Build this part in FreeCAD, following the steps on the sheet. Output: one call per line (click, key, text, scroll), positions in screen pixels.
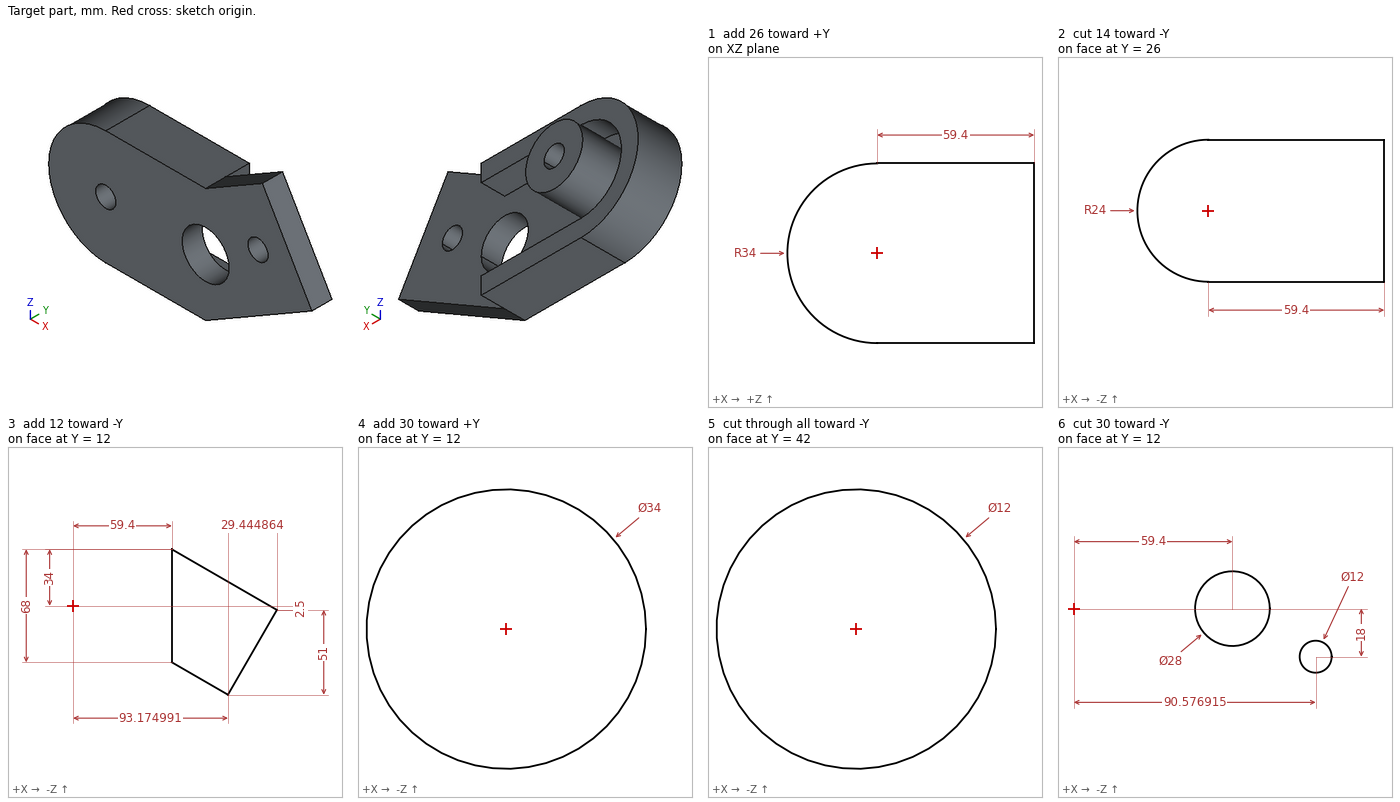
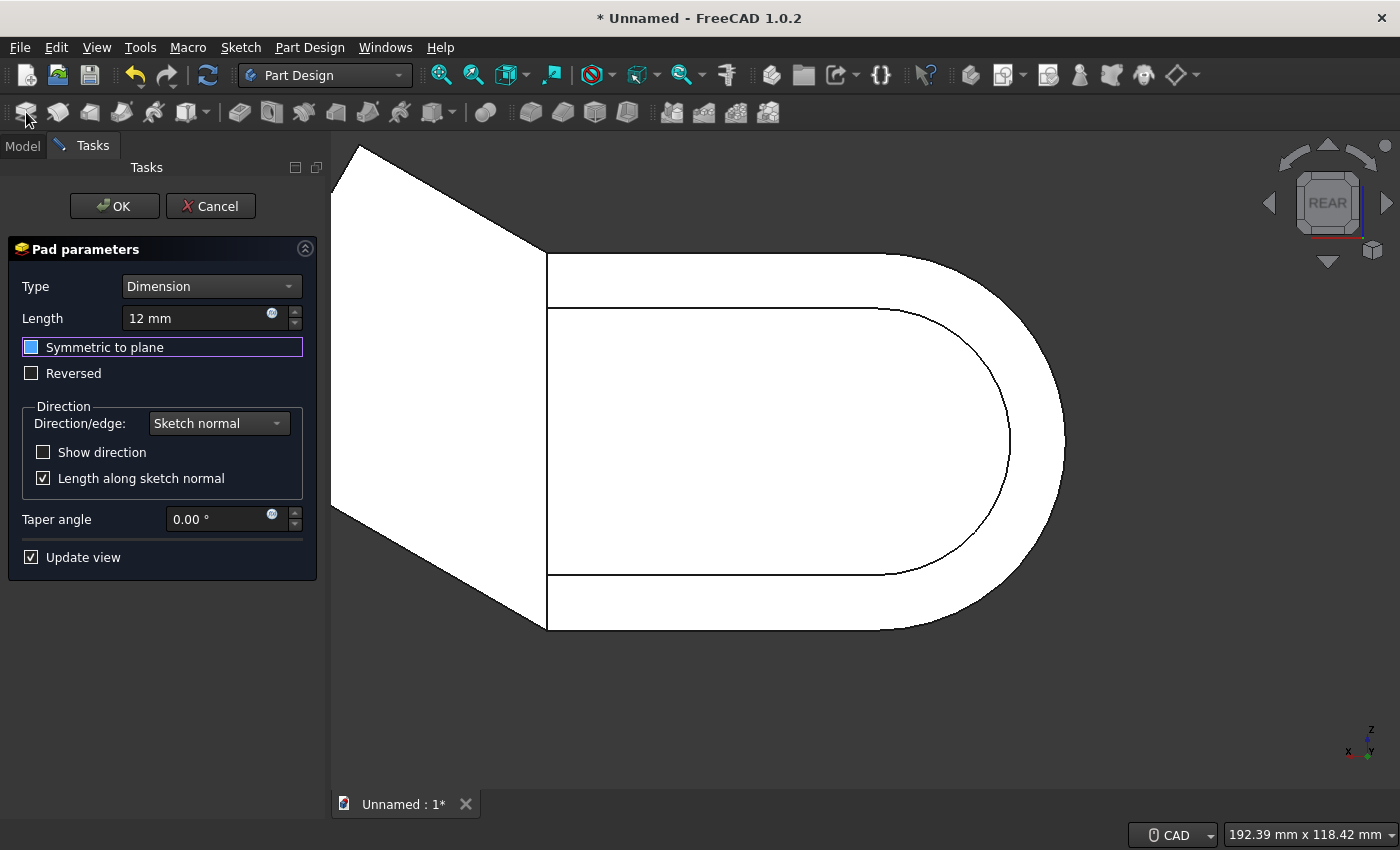
click(30, 373)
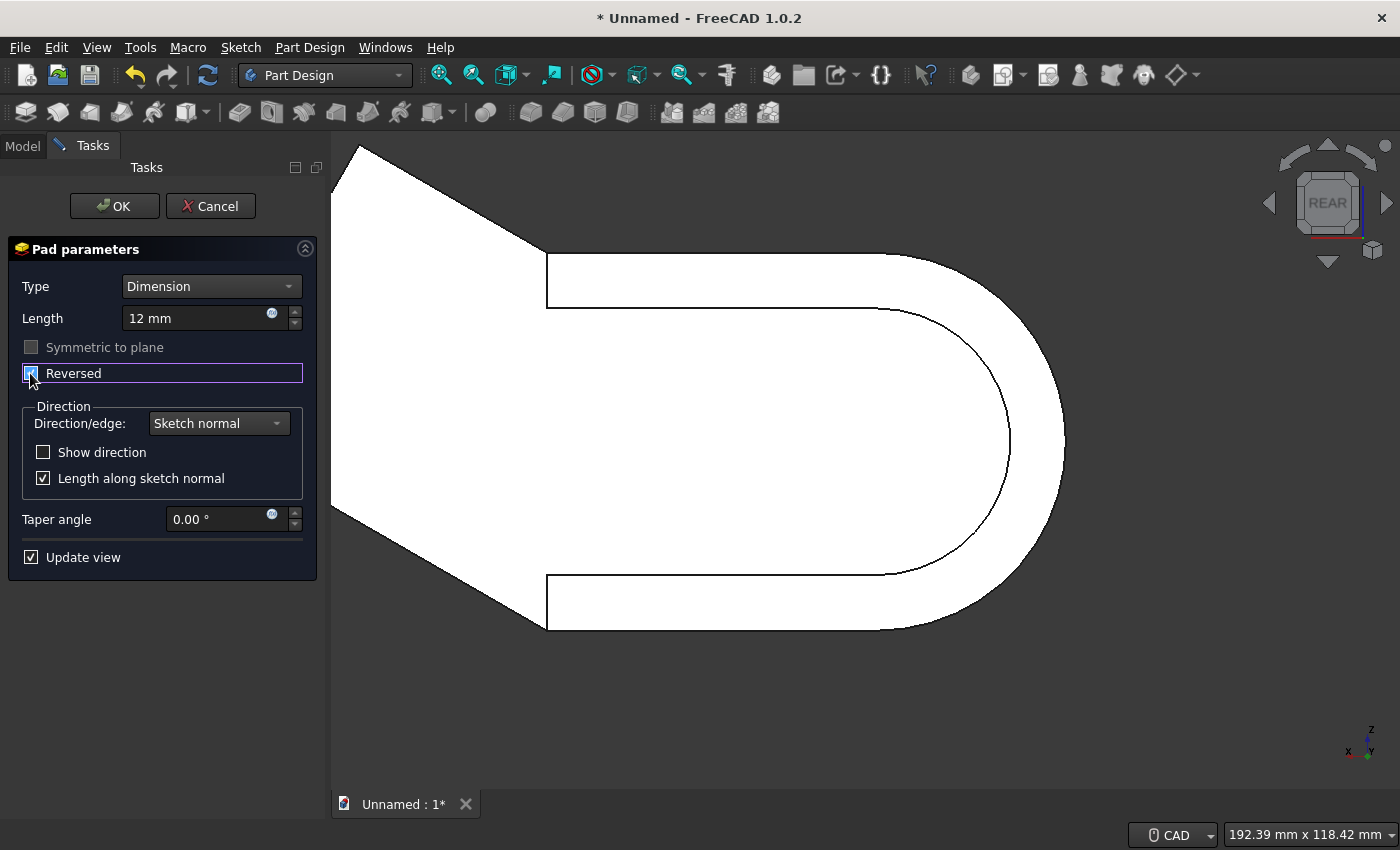
click(115, 206)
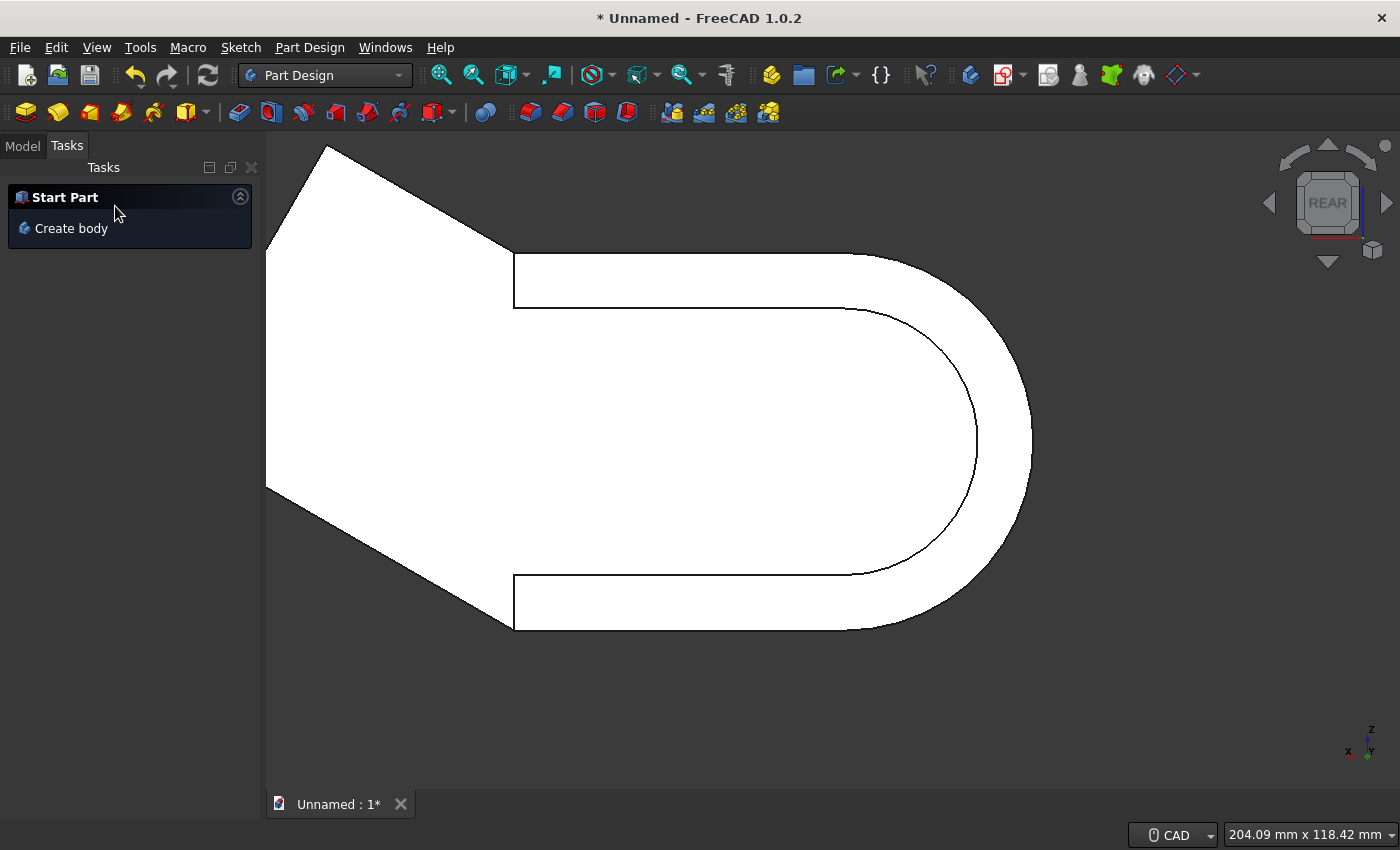
click(442, 76)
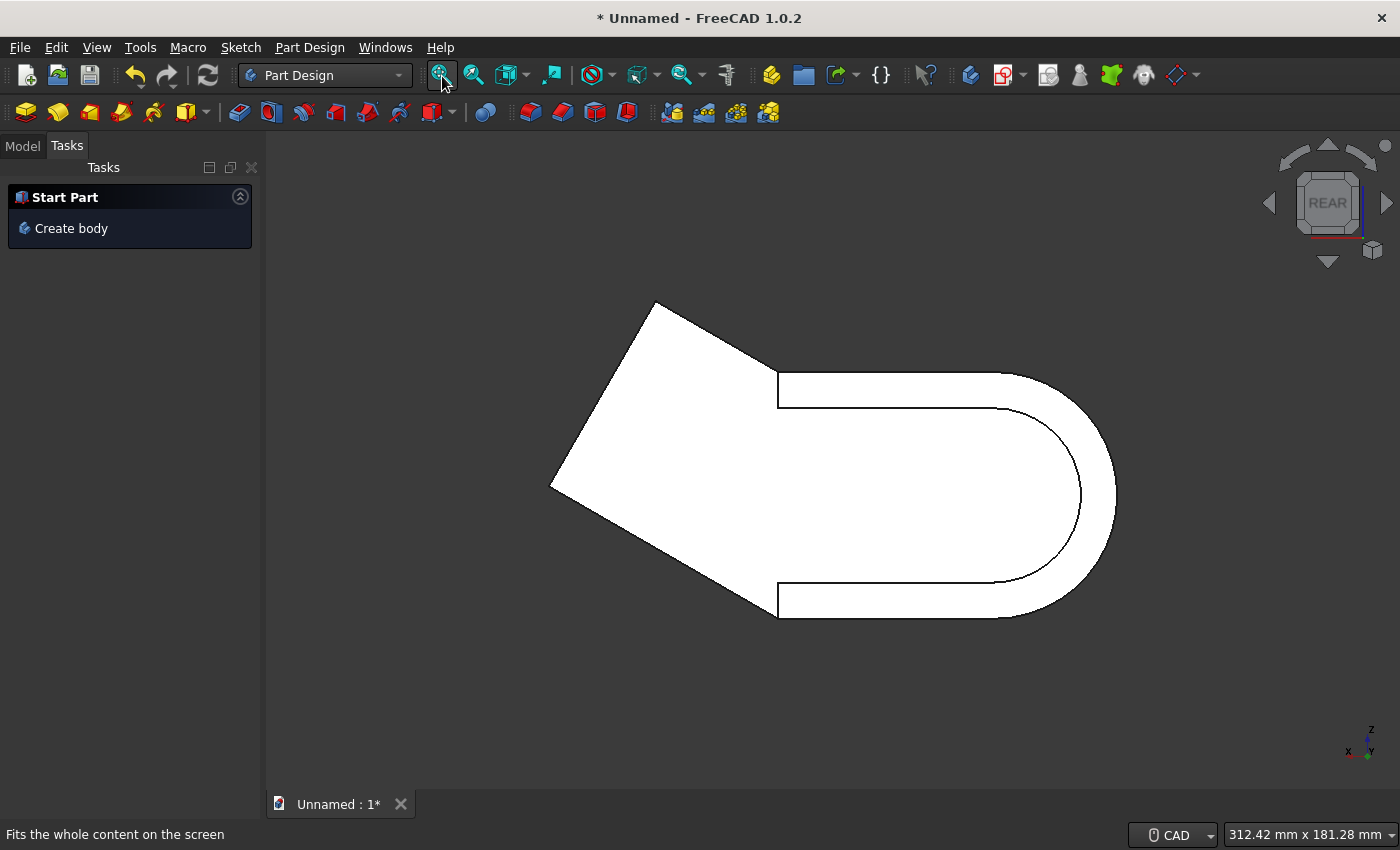
click(663, 459)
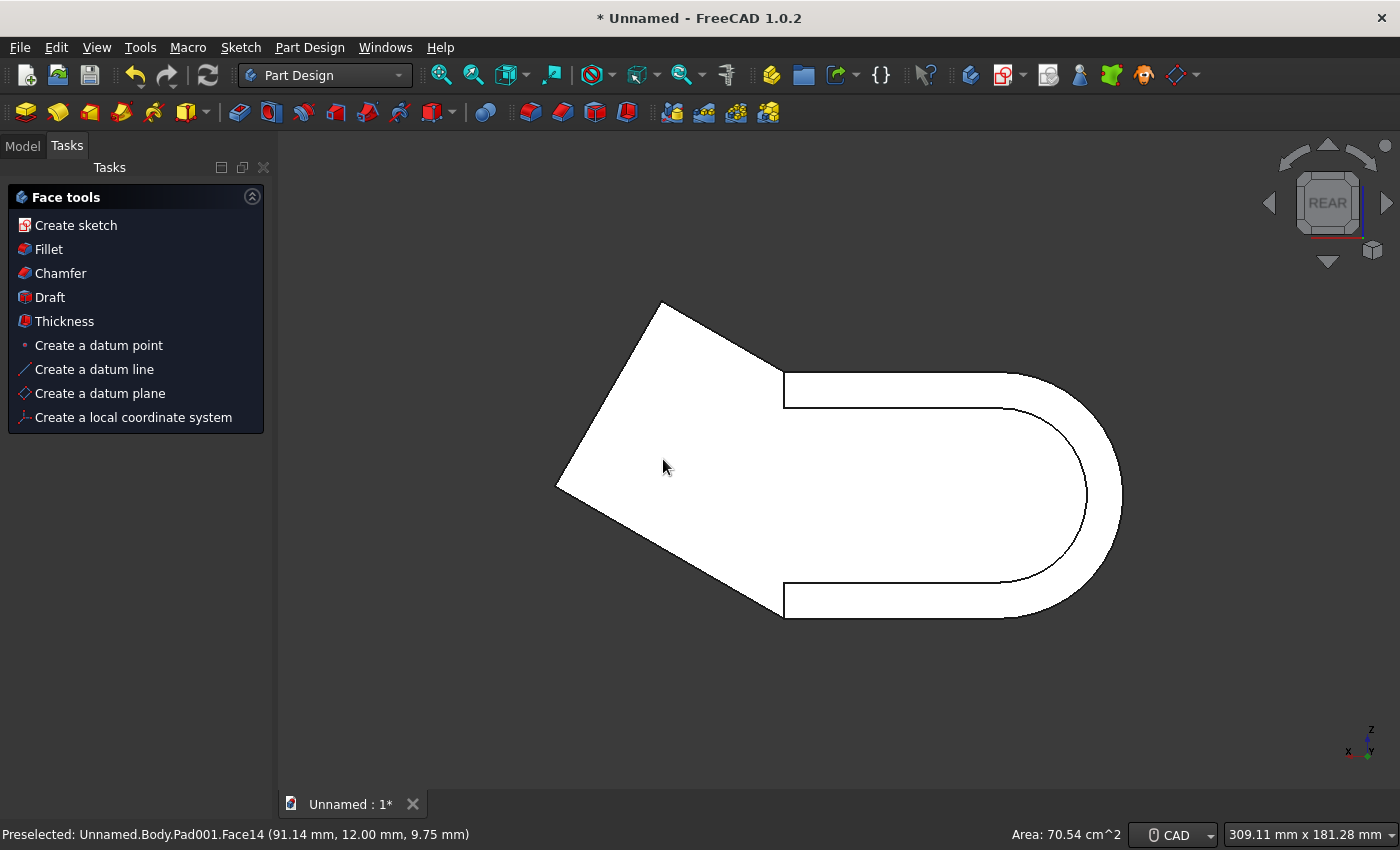
click(1004, 76)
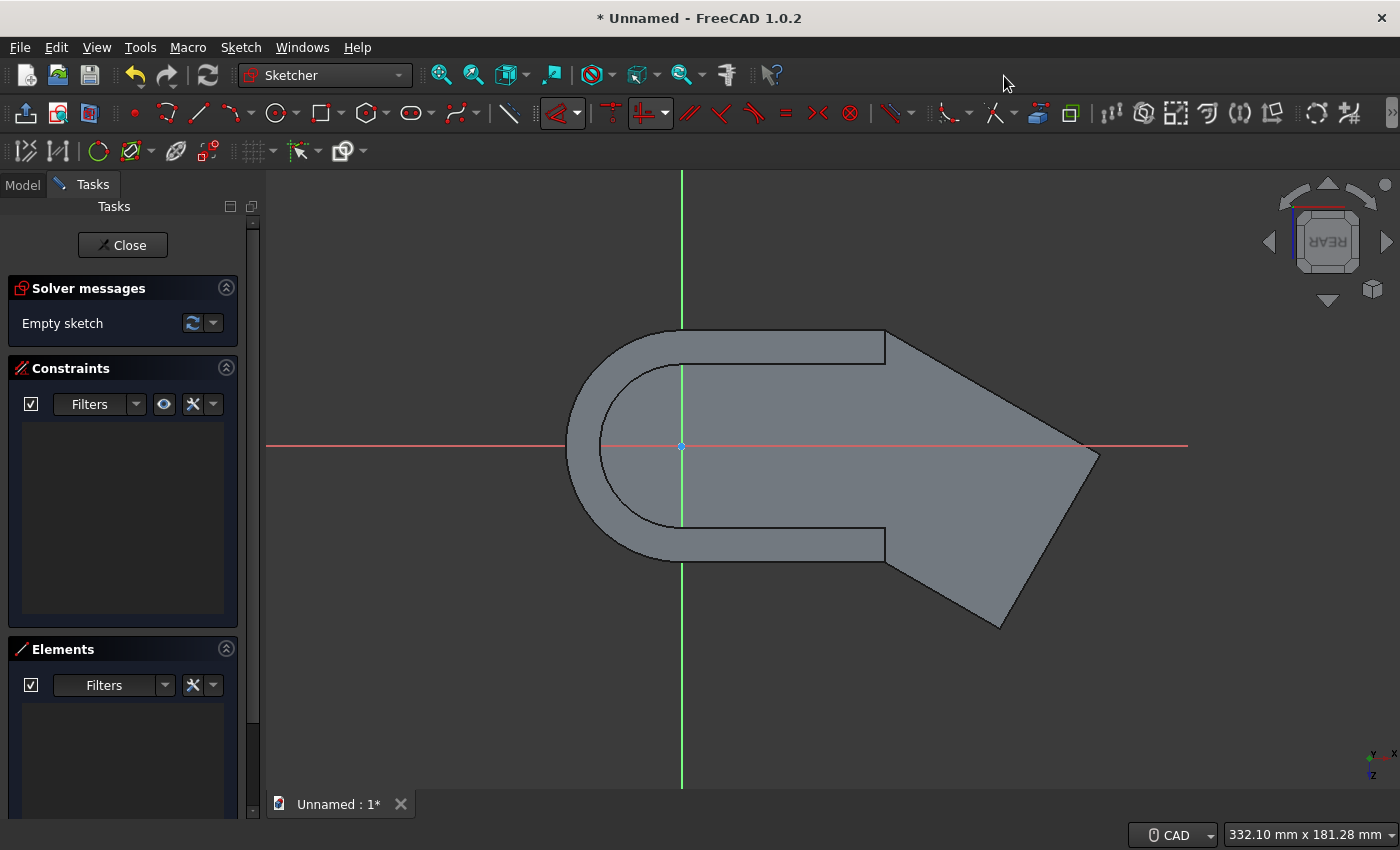
click(90, 114)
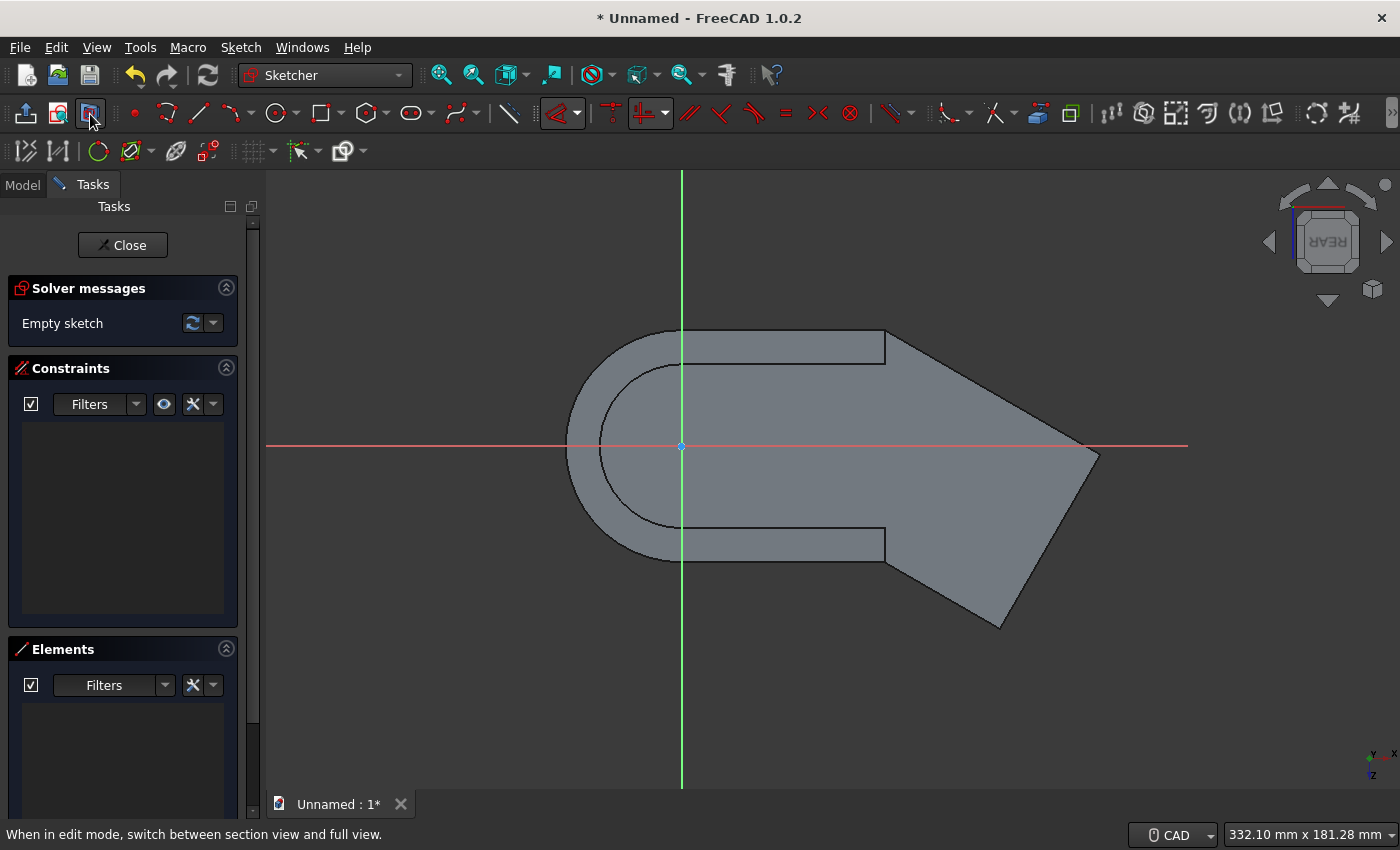
scroll(646, 432, up, 6)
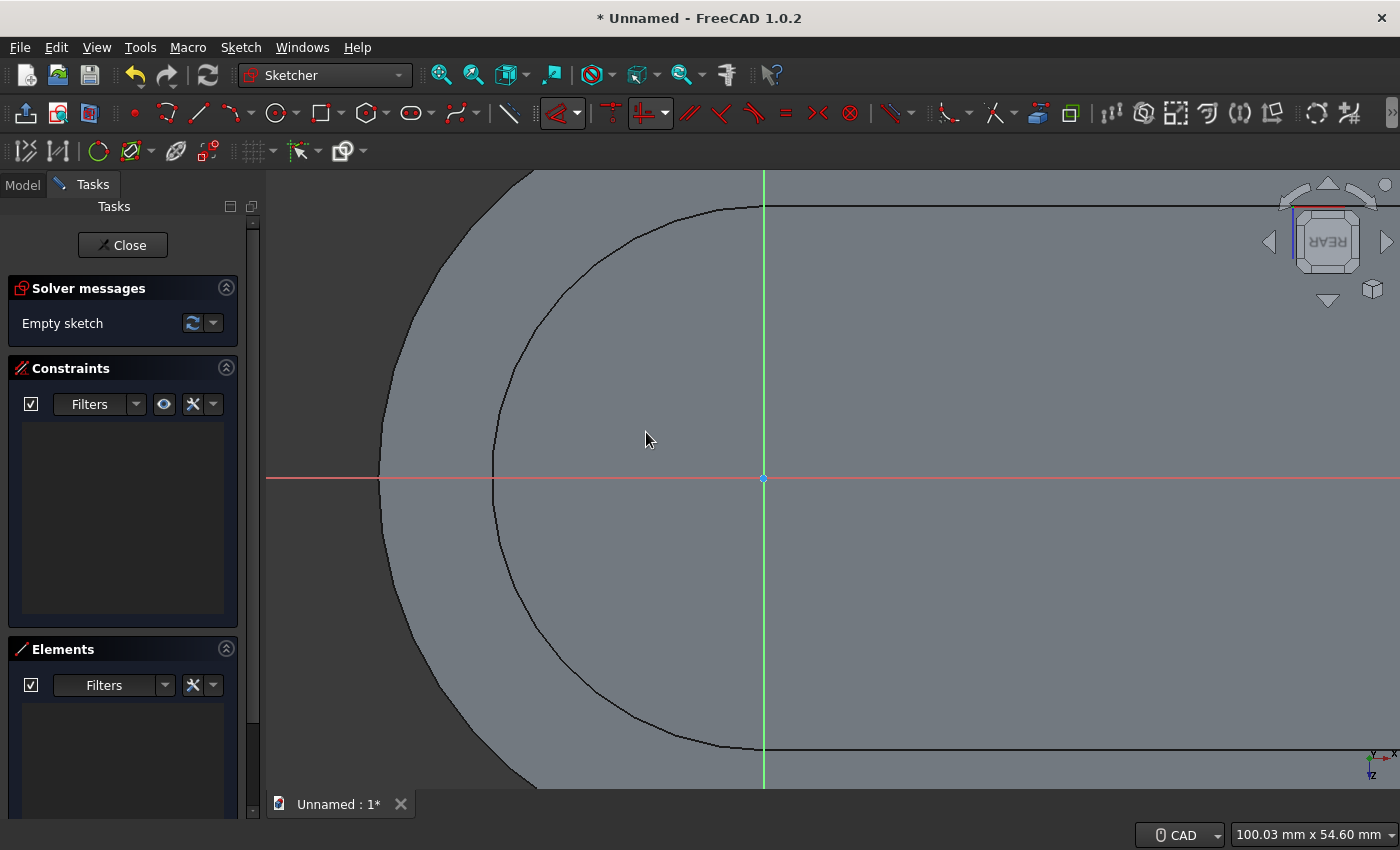
click(276, 114)